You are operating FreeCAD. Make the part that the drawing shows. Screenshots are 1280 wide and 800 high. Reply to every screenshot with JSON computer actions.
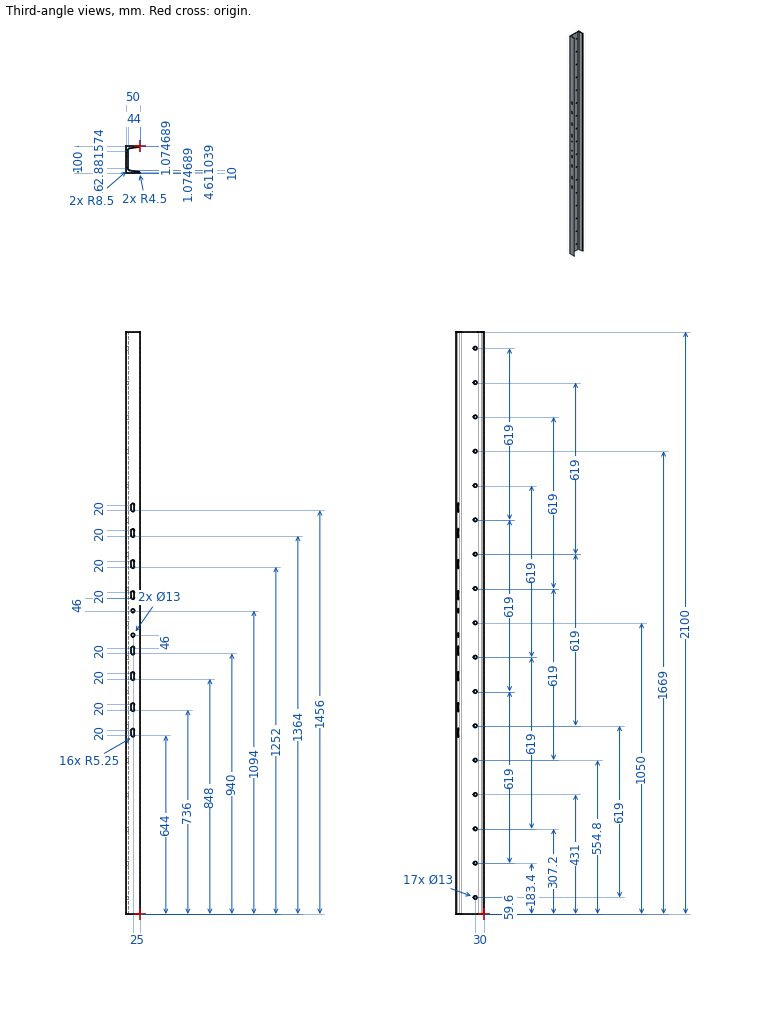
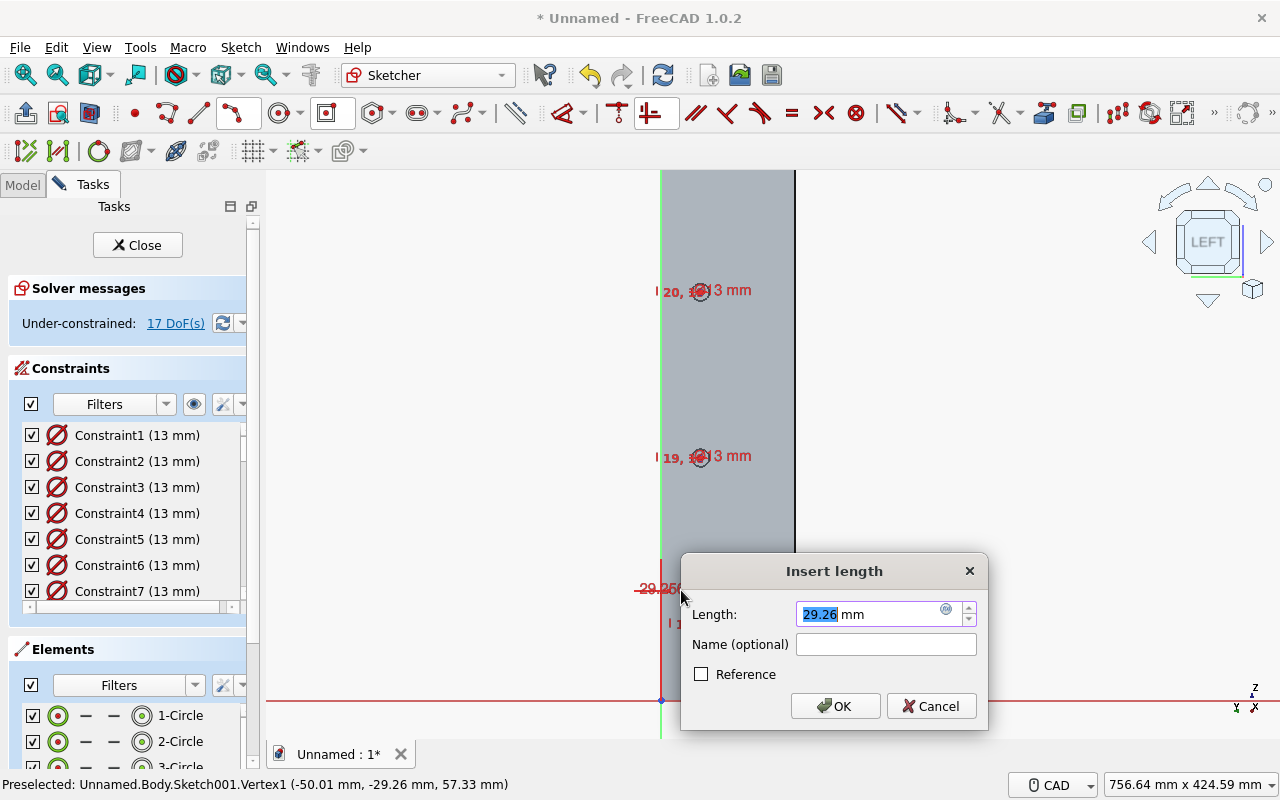
{"action": "type", "text": "30"}
{"action": "key", "text": "Return"}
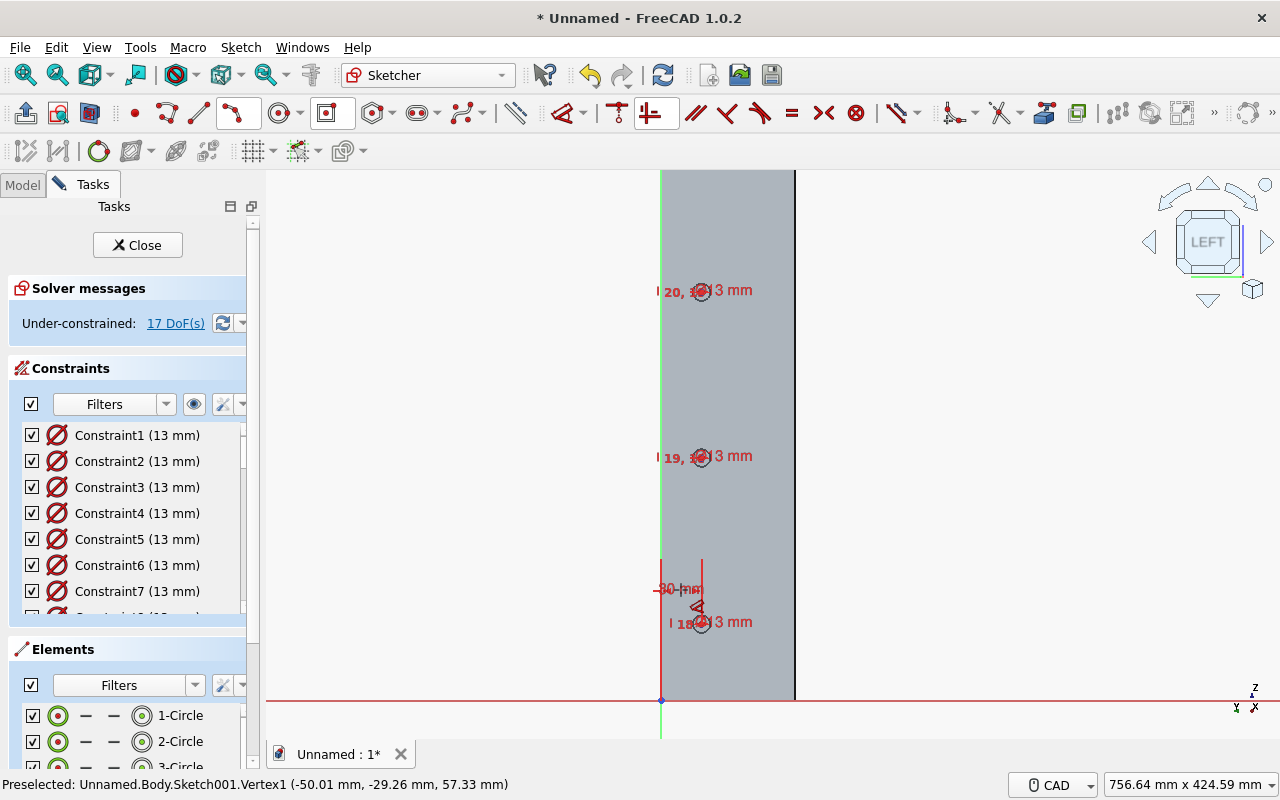
{"action": "scroll", "coordinate": [707, 631], "scroll_direction": "down", "scroll_amount": 10}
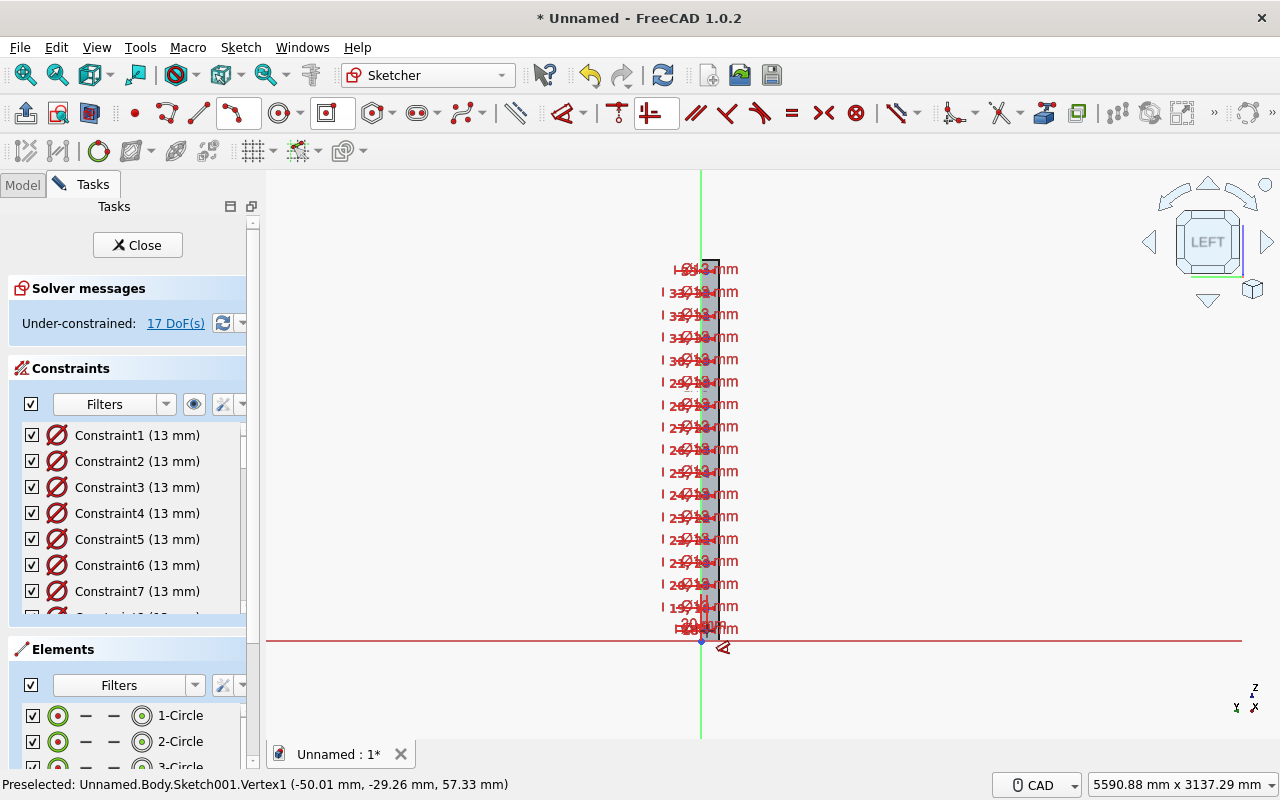
{"action": "left_click", "coordinate": [707, 563]}
{"action": "left_click", "coordinate": [667, 602]}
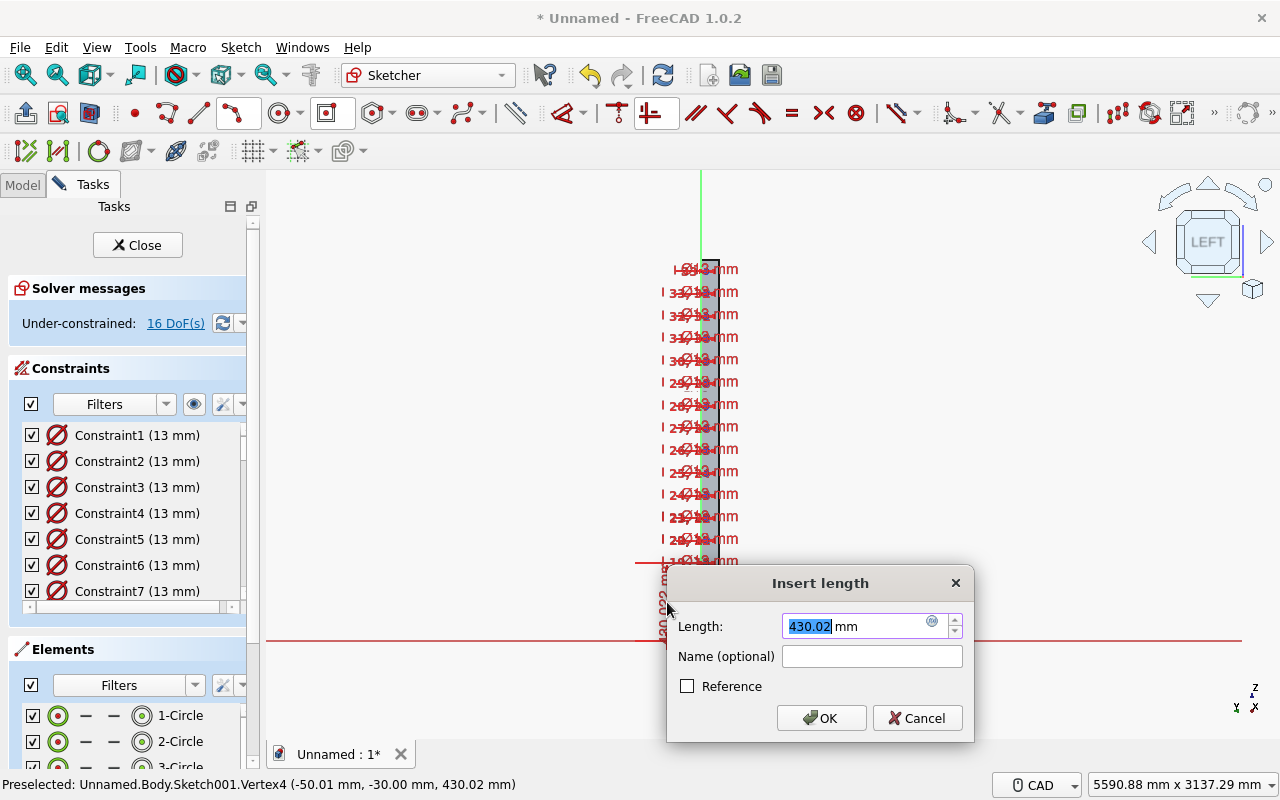
{"action": "type", "text": "431"}
{"action": "key", "text": "Return"}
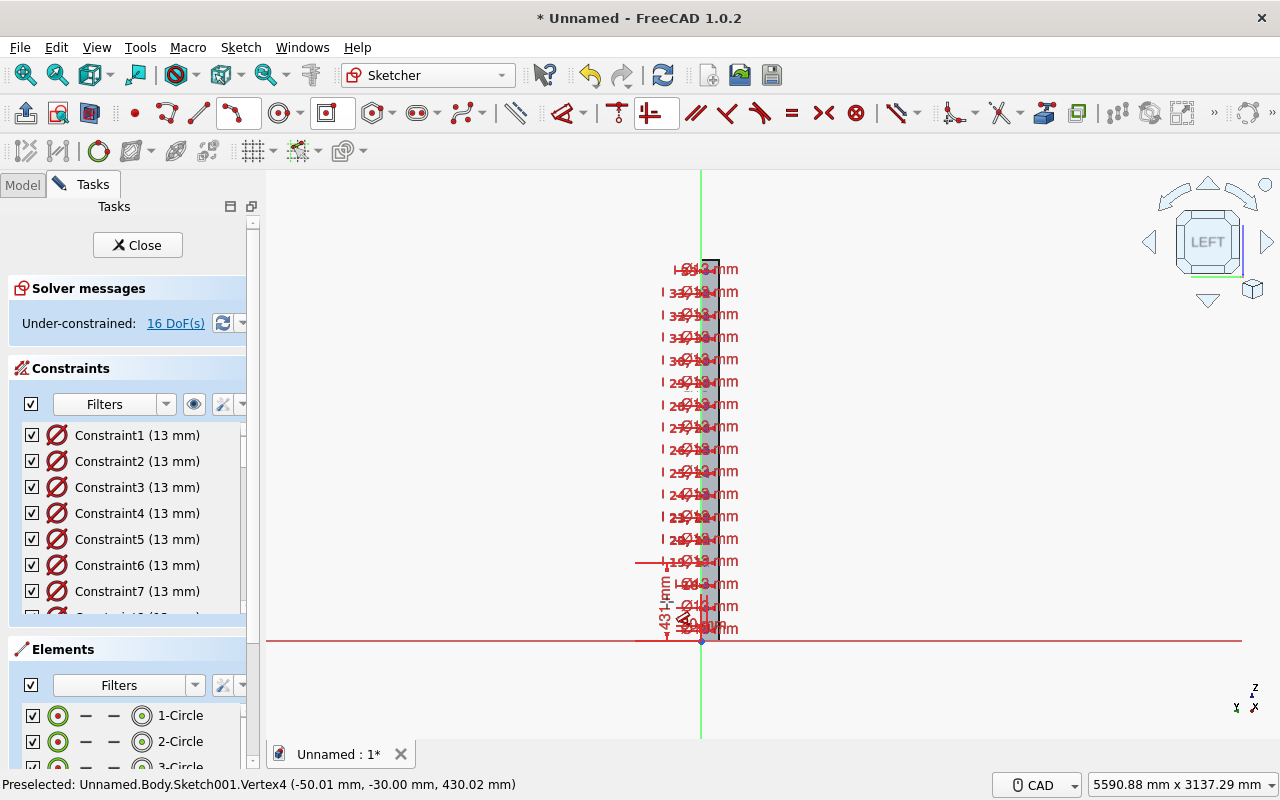
{"action": "scroll", "coordinate": [707, 631], "scroll_direction": "up", "scroll_amount": 7}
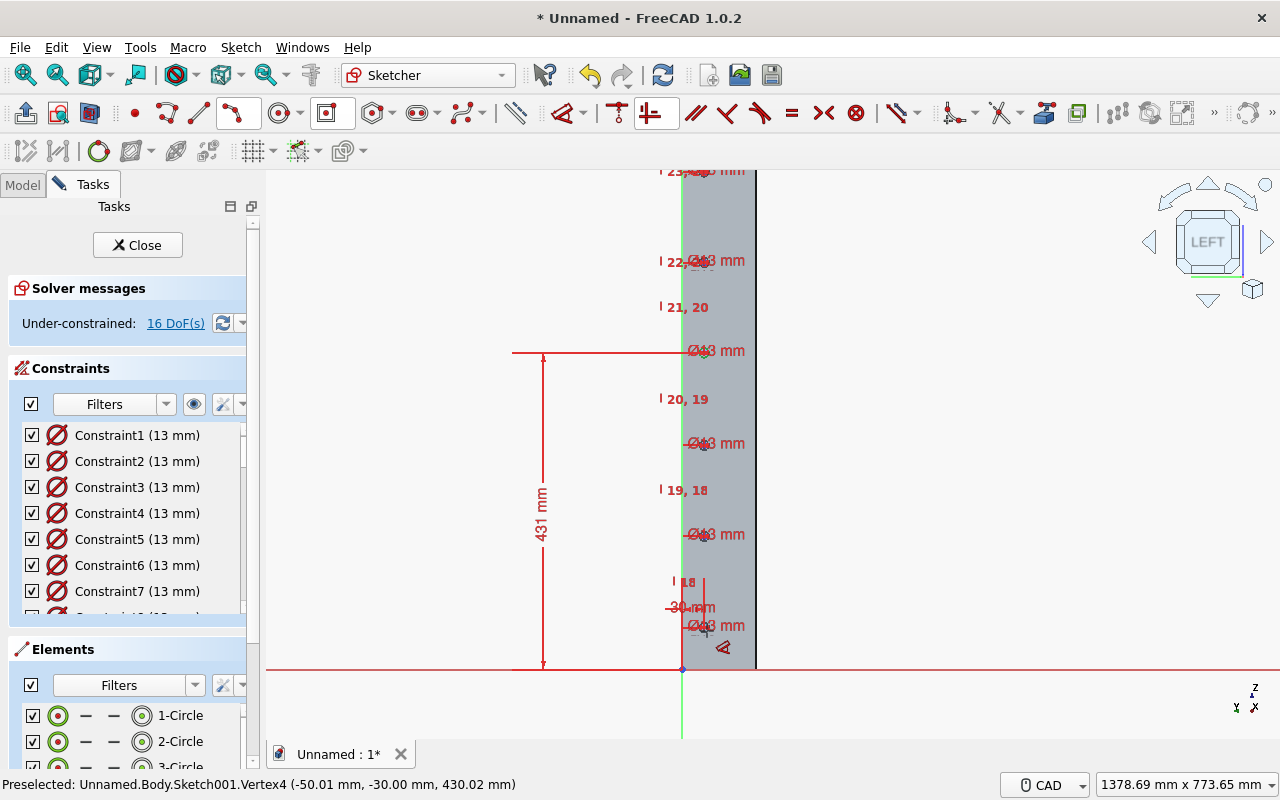
{"action": "left_click", "coordinate": [704, 628]}
{"action": "left_click", "coordinate": [648, 649]}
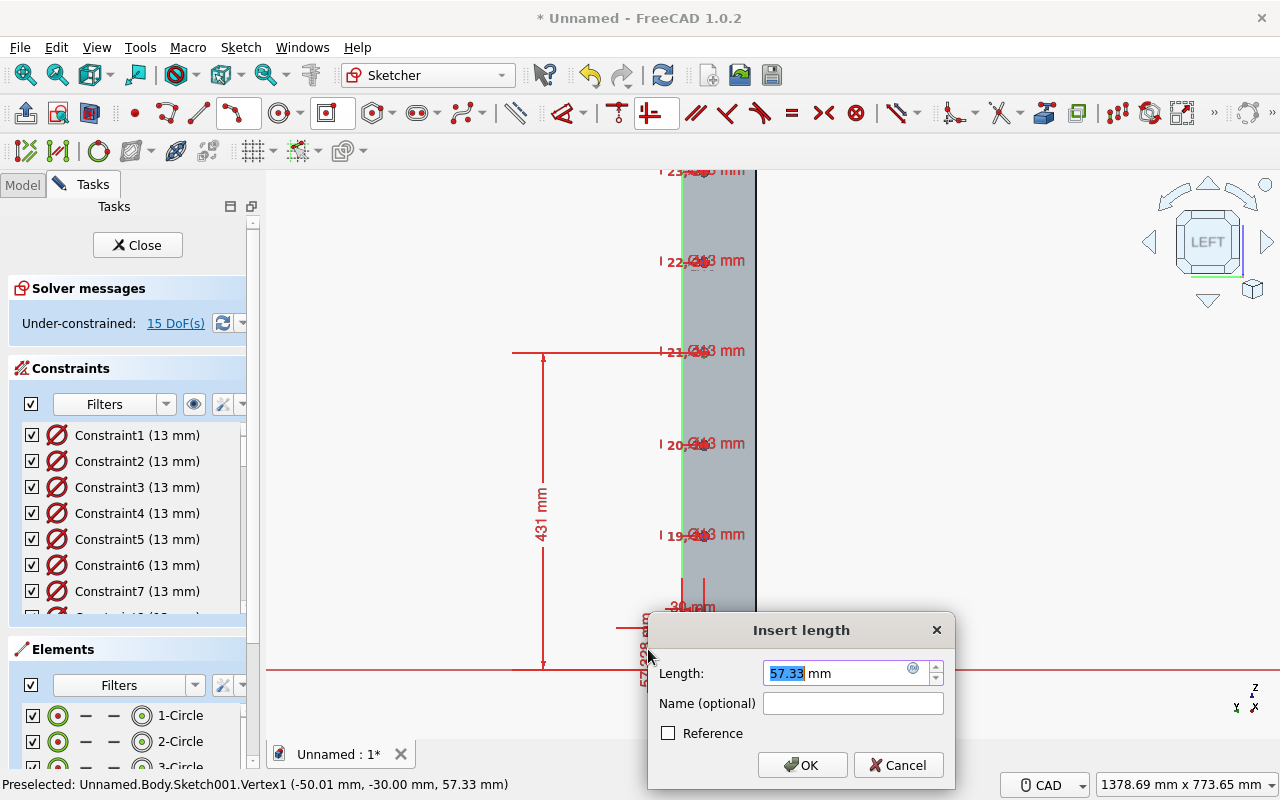
{"action": "type", "text": "59.6"}
{"action": "key", "text": "Return"}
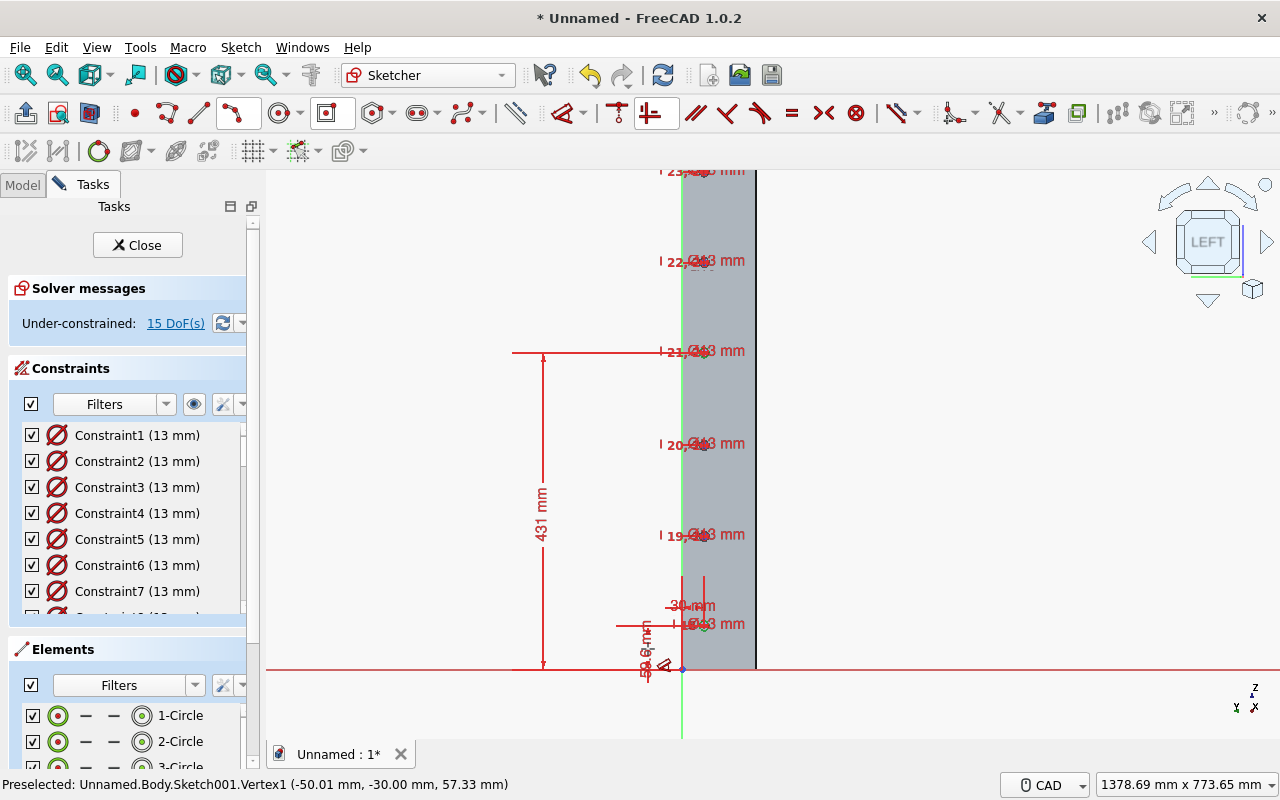
{"action": "scroll", "coordinate": [707, 630], "scroll_direction": "down", "scroll_amount": 7}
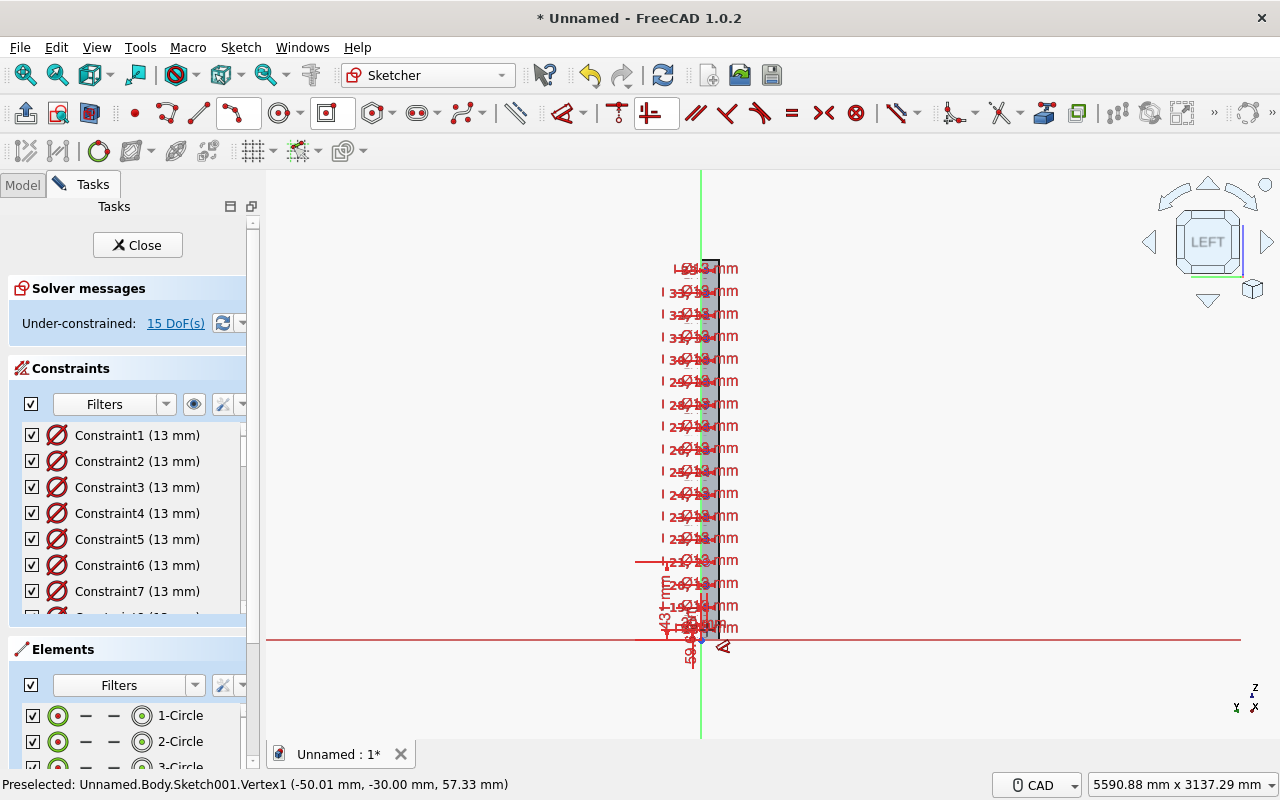
{"action": "left_click", "coordinate": [707, 450]}
{"action": "left_click", "coordinate": [667, 545]}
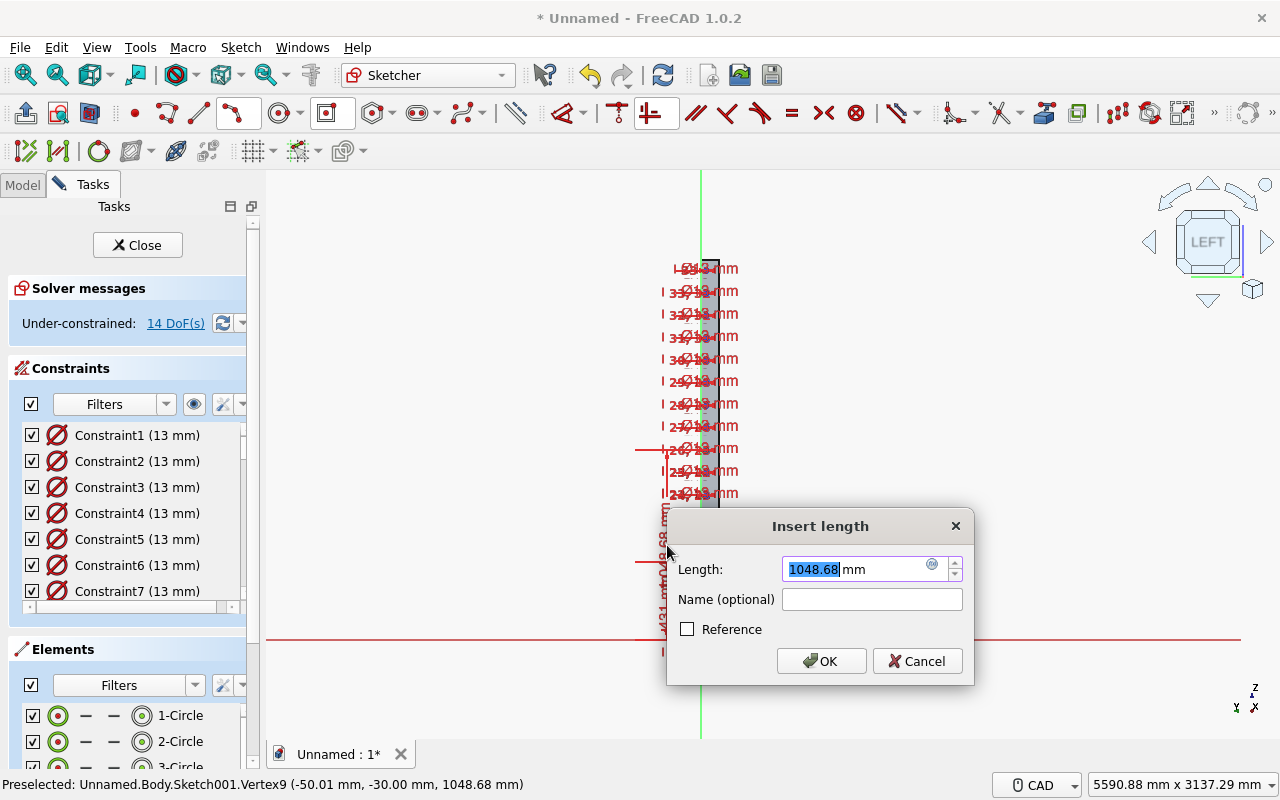
{"action": "type", "text": "1050"}
{"action": "key", "text": "Return"}